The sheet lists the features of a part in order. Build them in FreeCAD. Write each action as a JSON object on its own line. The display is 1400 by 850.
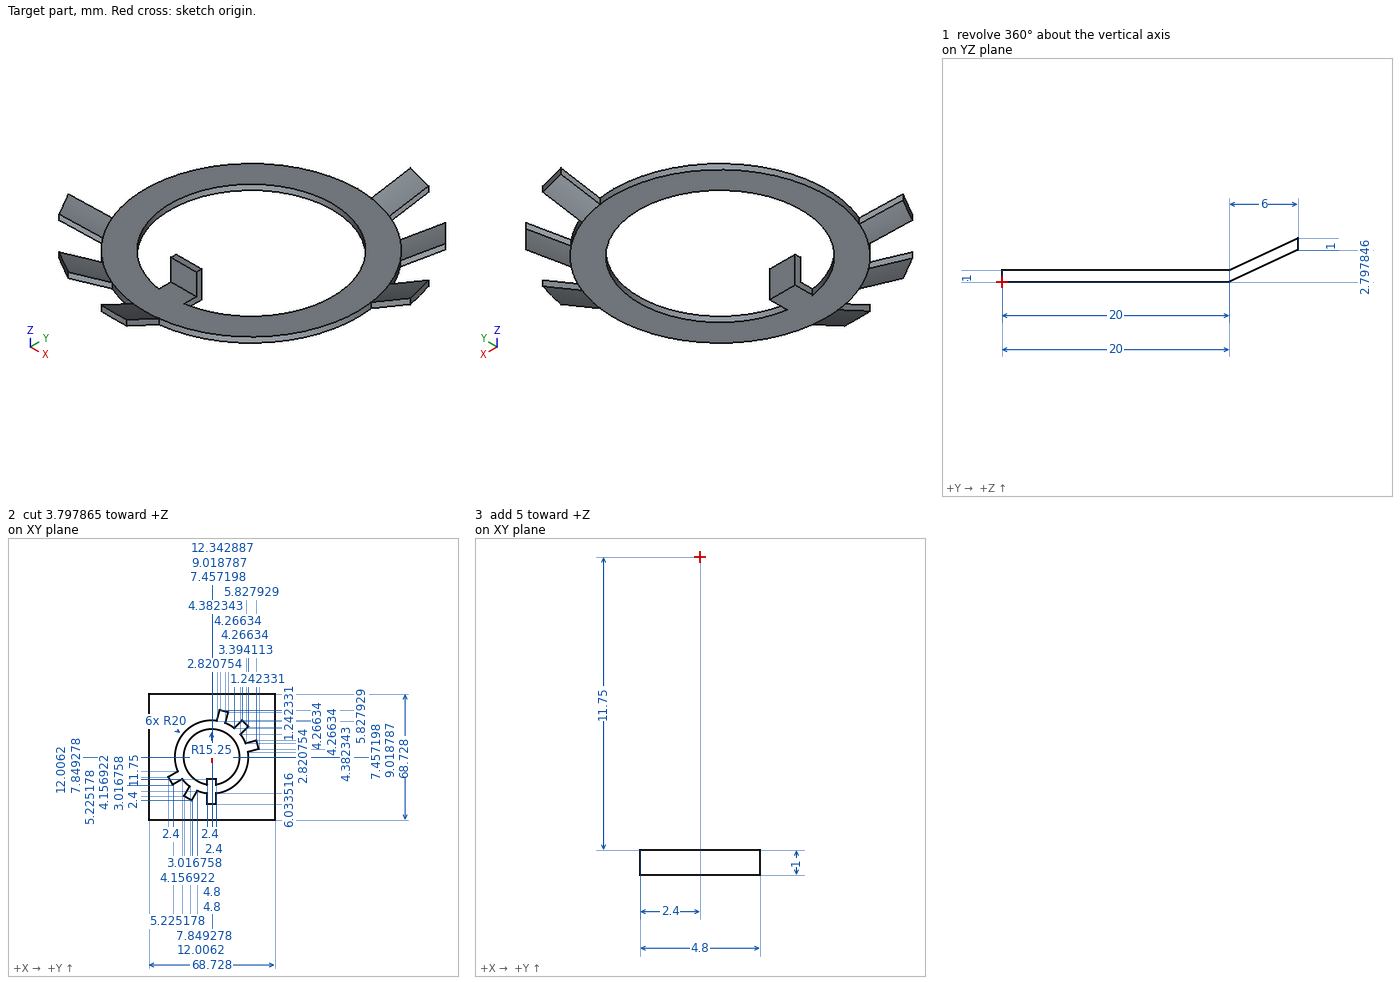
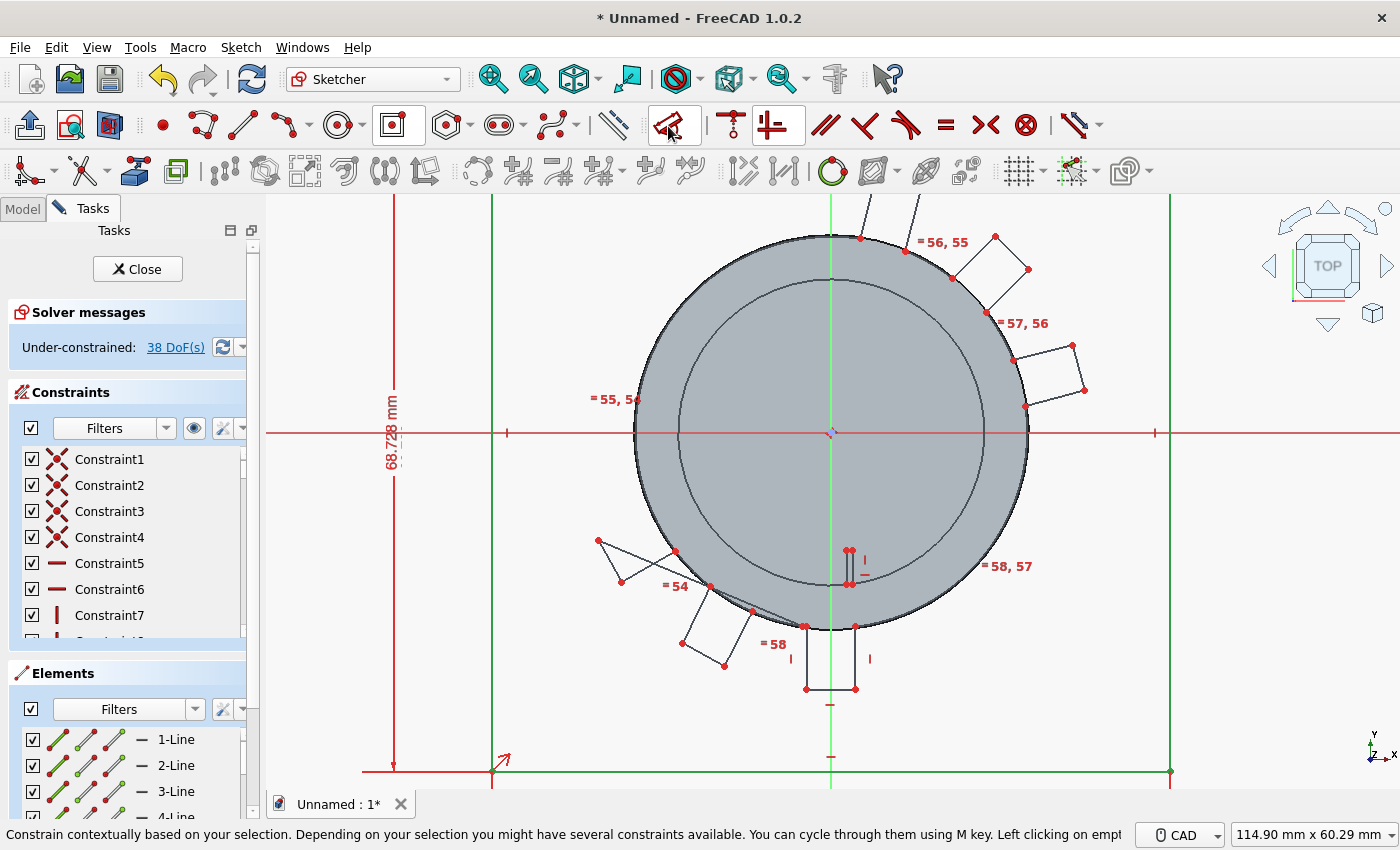
{"action": "left_click", "coordinate": [970, 367]}
{"action": "left_click", "coordinate": [1042, 333]}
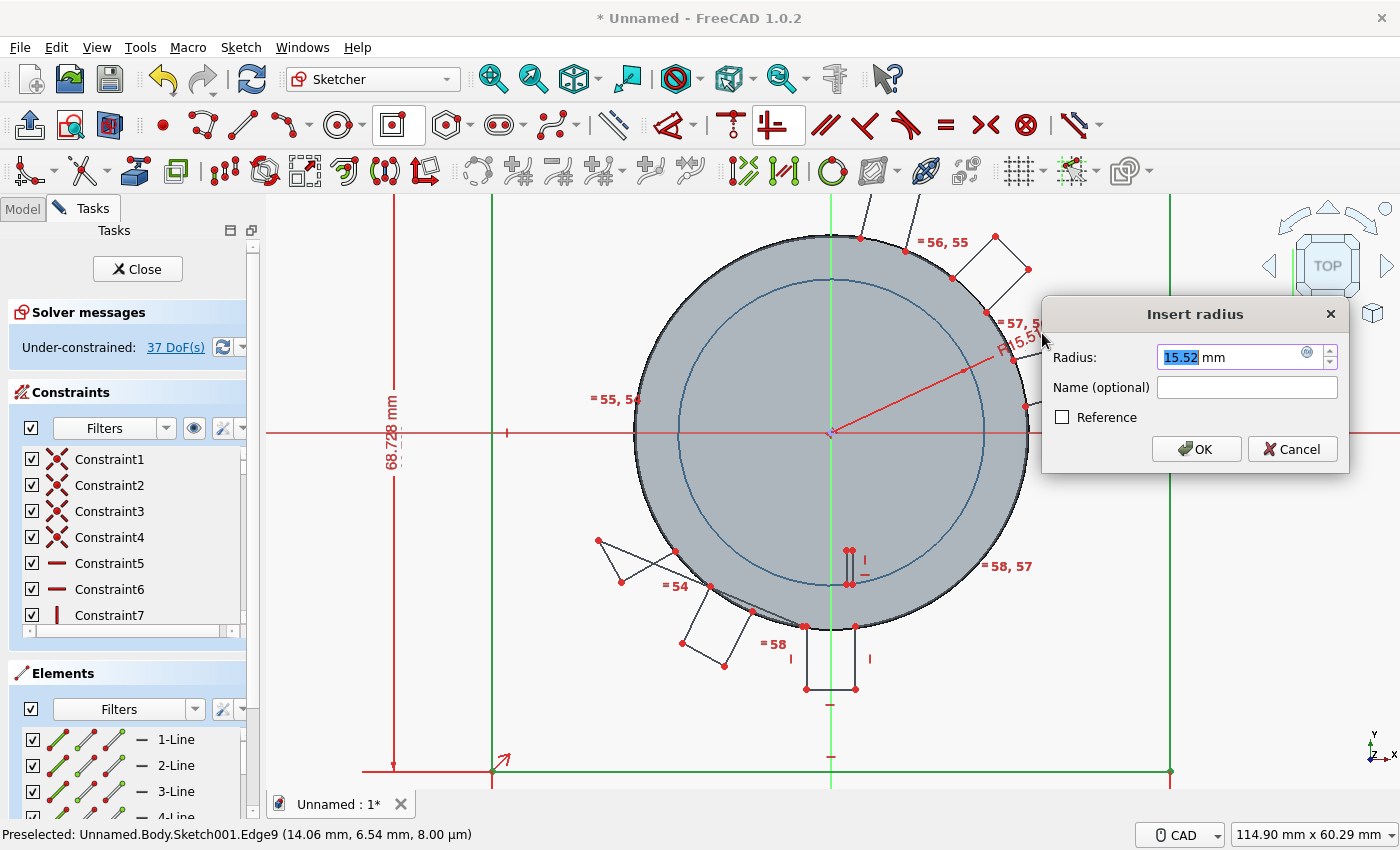
{"action": "type", "text": "15.25"}
{"action": "key", "text": "Return"}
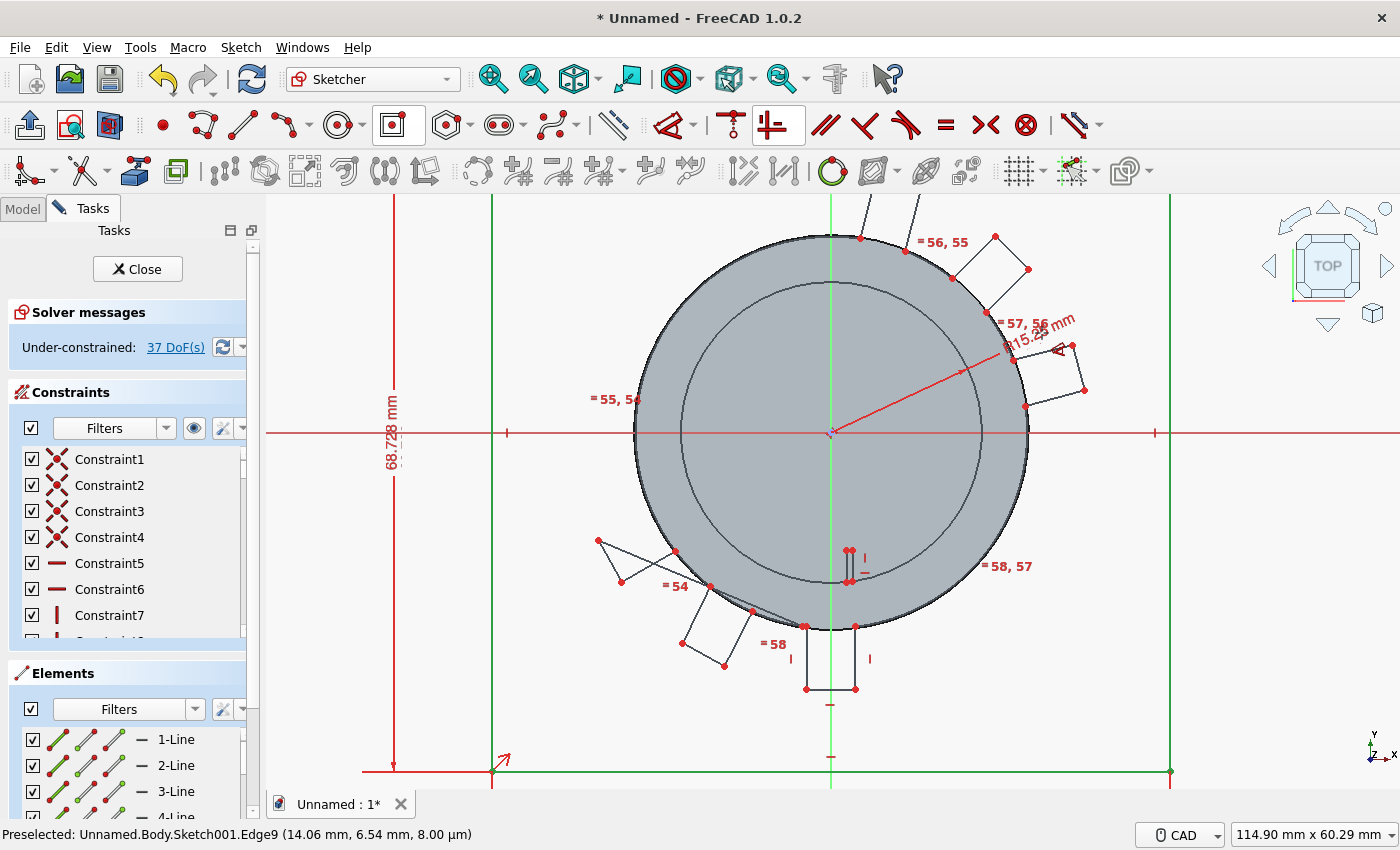
{"action": "scroll", "coordinate": [699, 577], "scroll_direction": "up", "scroll_amount": 11}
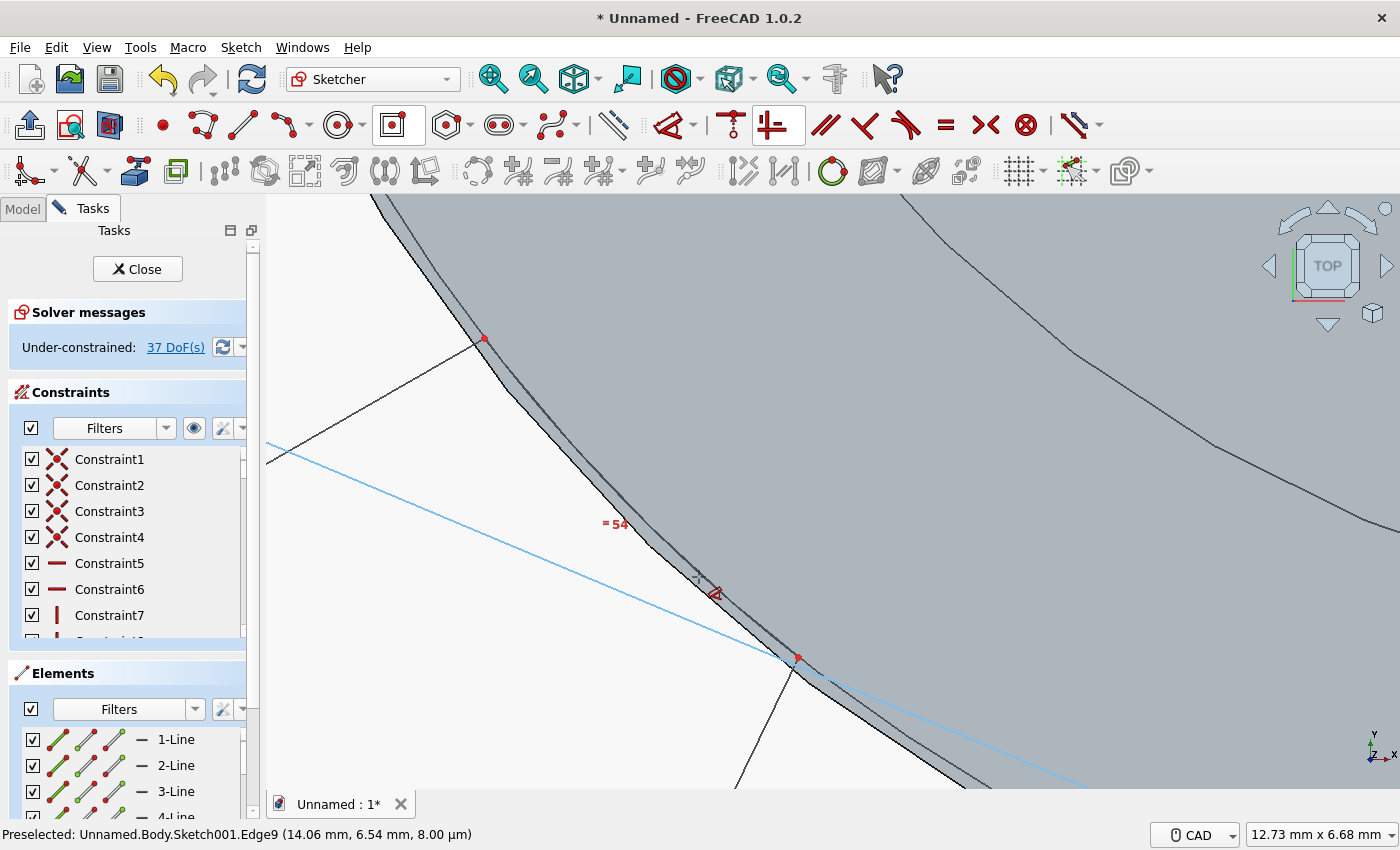
{"action": "left_click", "coordinate": [696, 570]}
{"action": "left_click", "coordinate": [674, 594]}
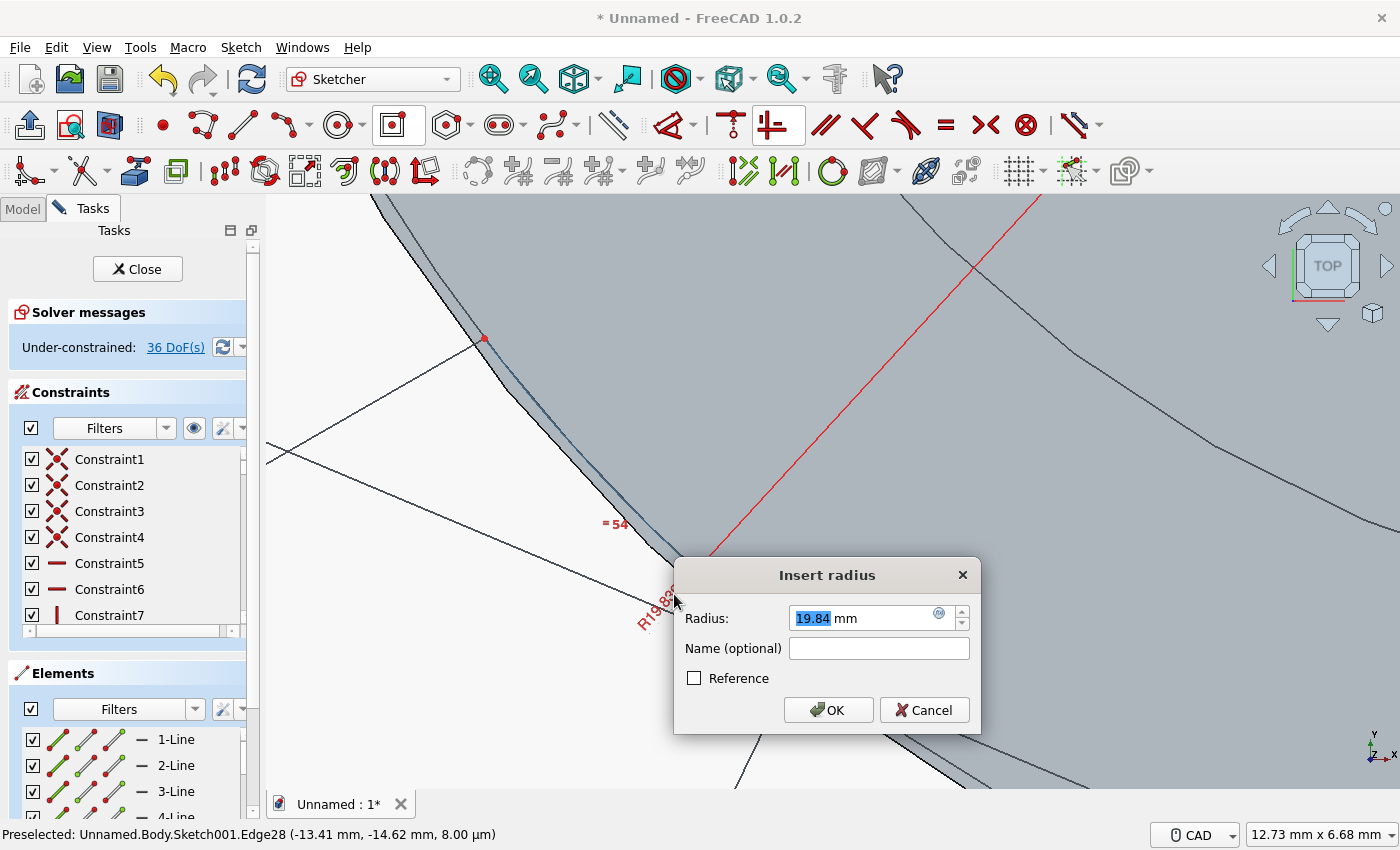
{"action": "type", "text": "20"}
{"action": "key", "text": "Return"}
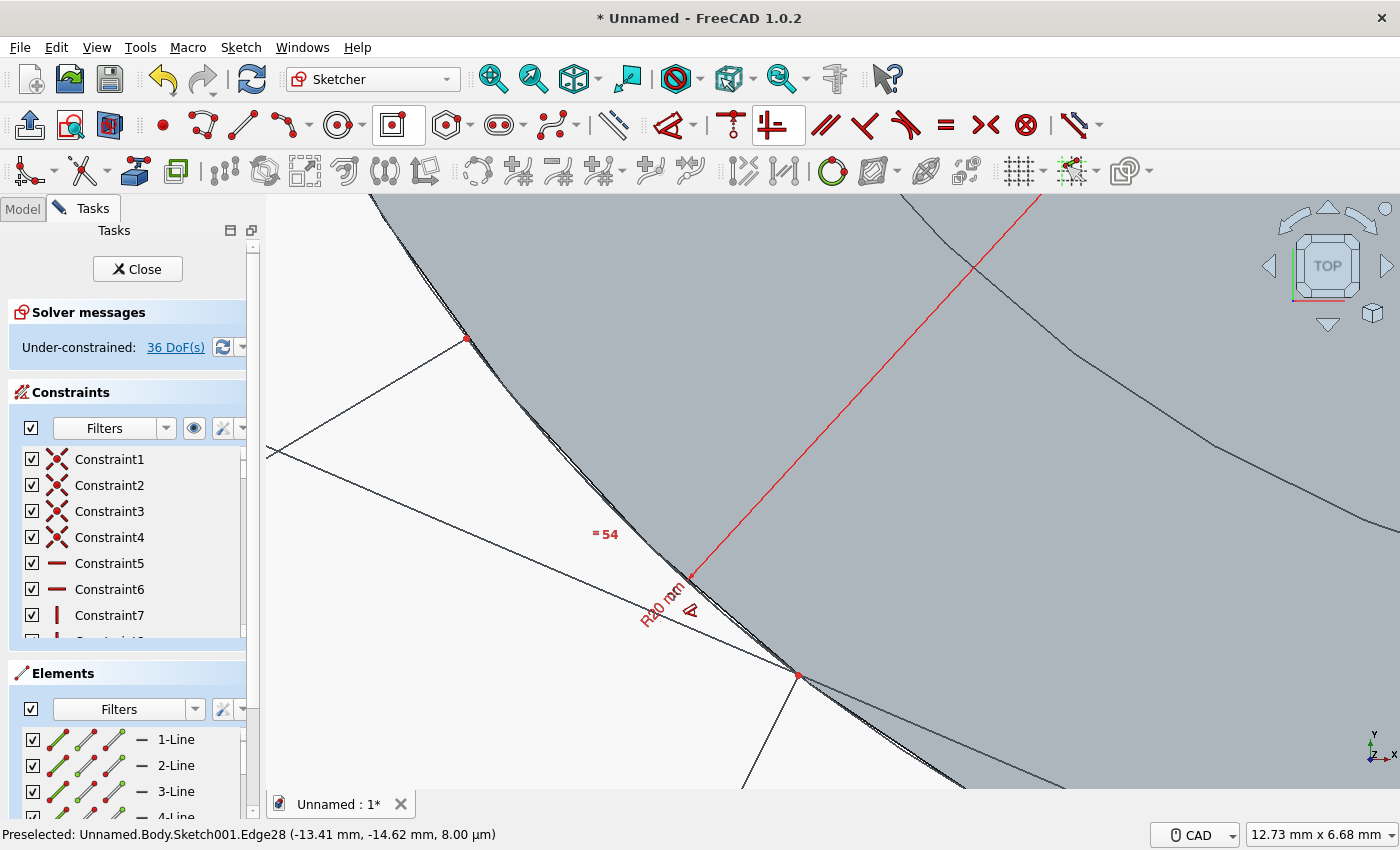
{"action": "scroll", "coordinate": [692, 571], "scroll_direction": "down", "scroll_amount": 14}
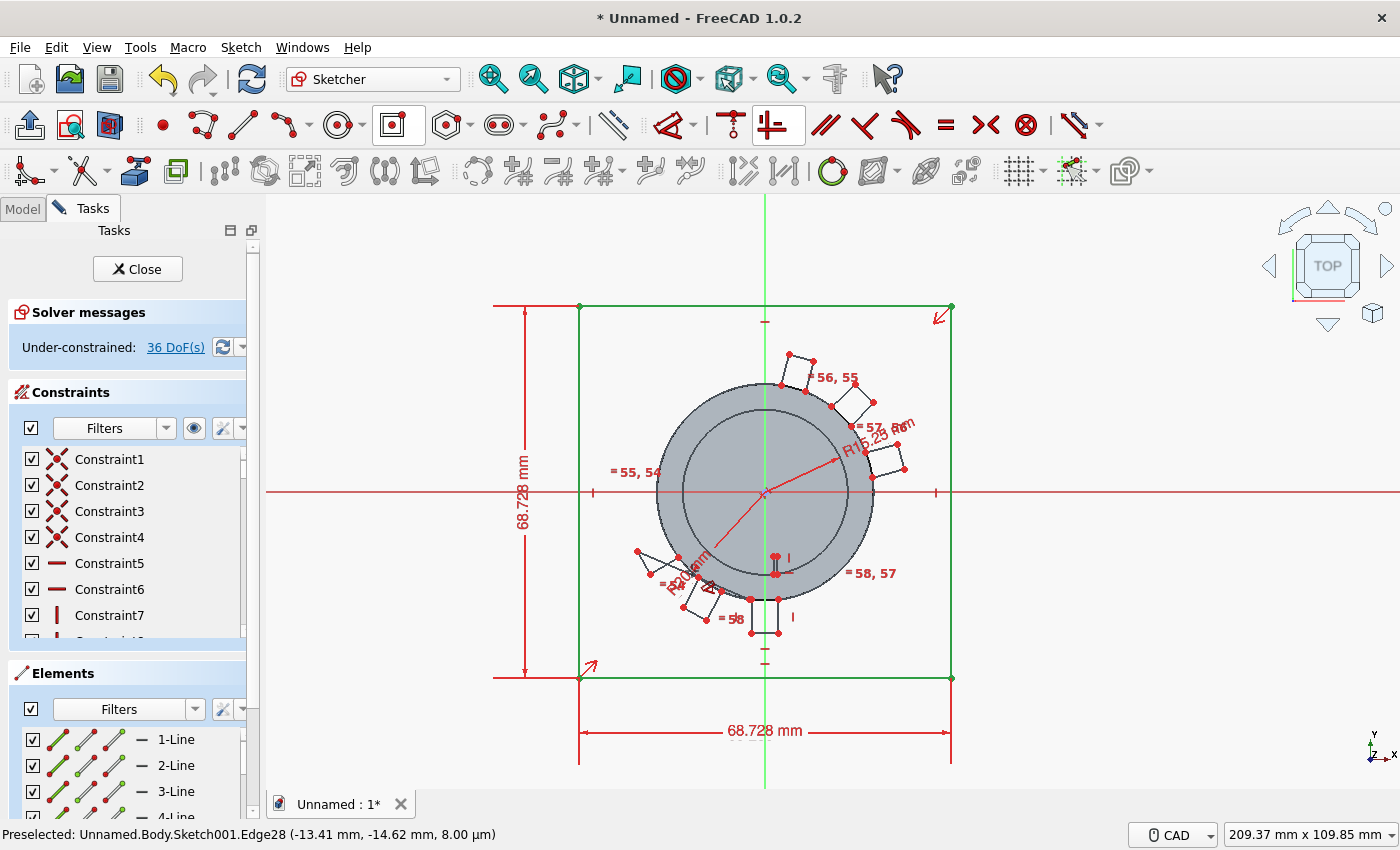
{"action": "scroll", "coordinate": [775, 557], "scroll_direction": "up", "scroll_amount": 14}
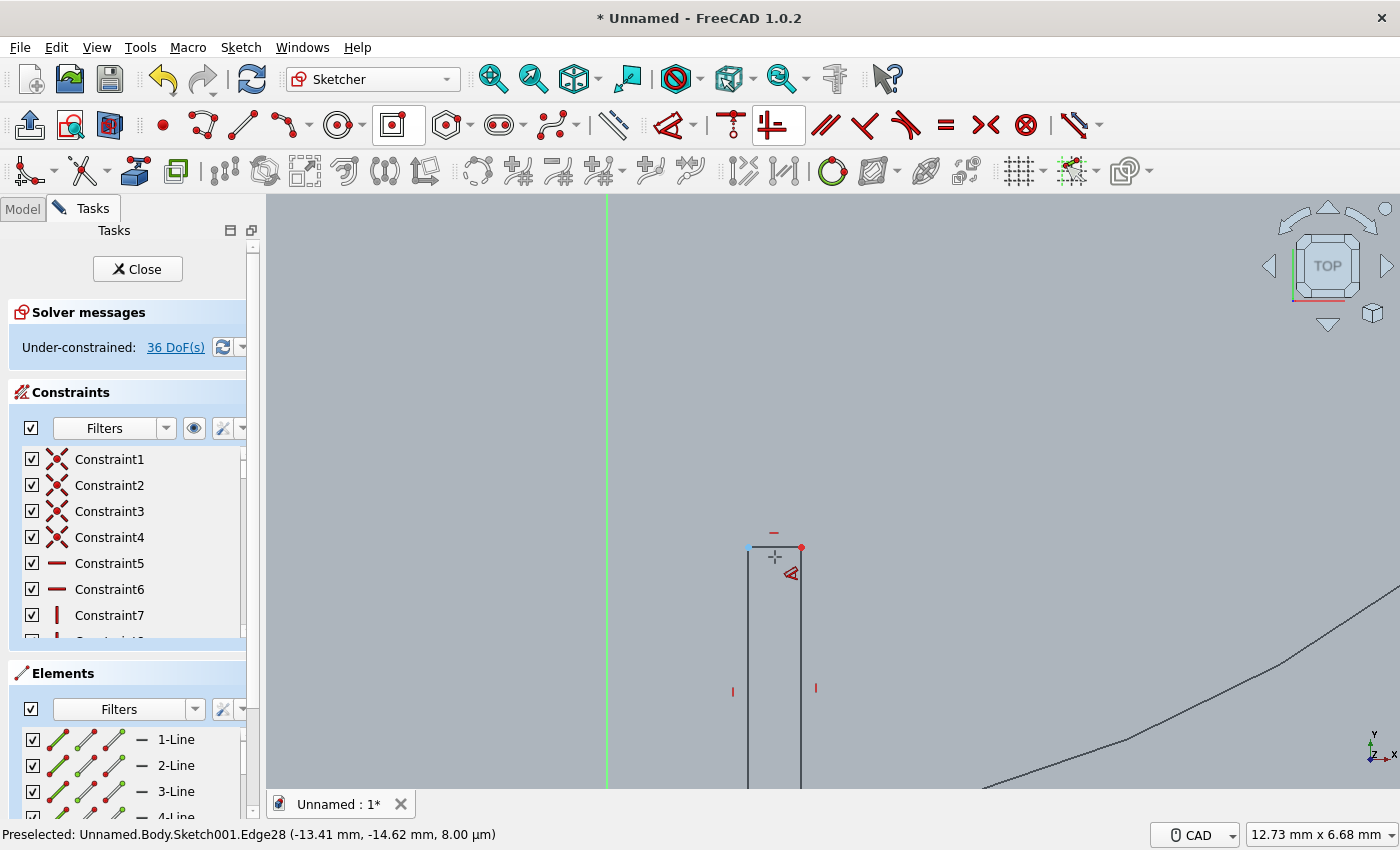
{"action": "left_click", "coordinate": [764, 547]}
{"action": "left_click", "coordinate": [775, 581]}